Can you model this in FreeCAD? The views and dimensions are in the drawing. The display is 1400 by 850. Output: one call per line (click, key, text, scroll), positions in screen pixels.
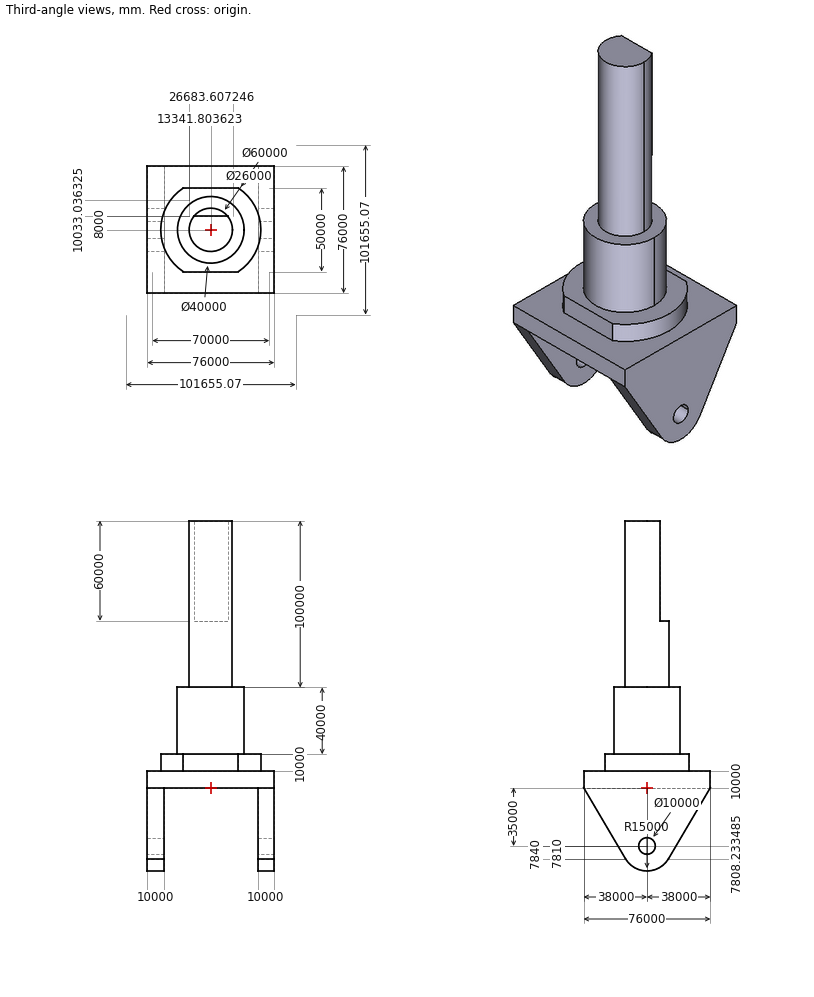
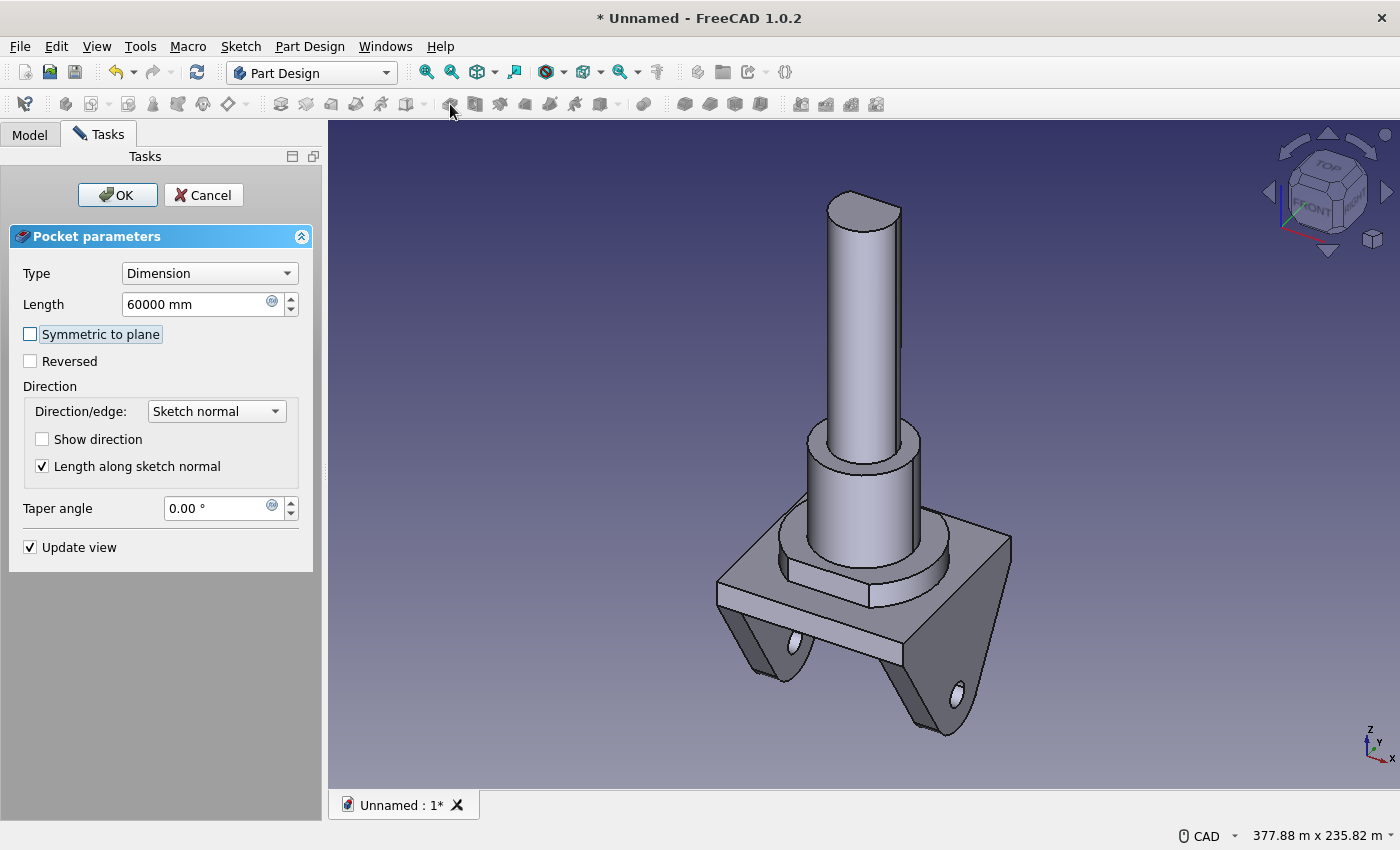
click(118, 195)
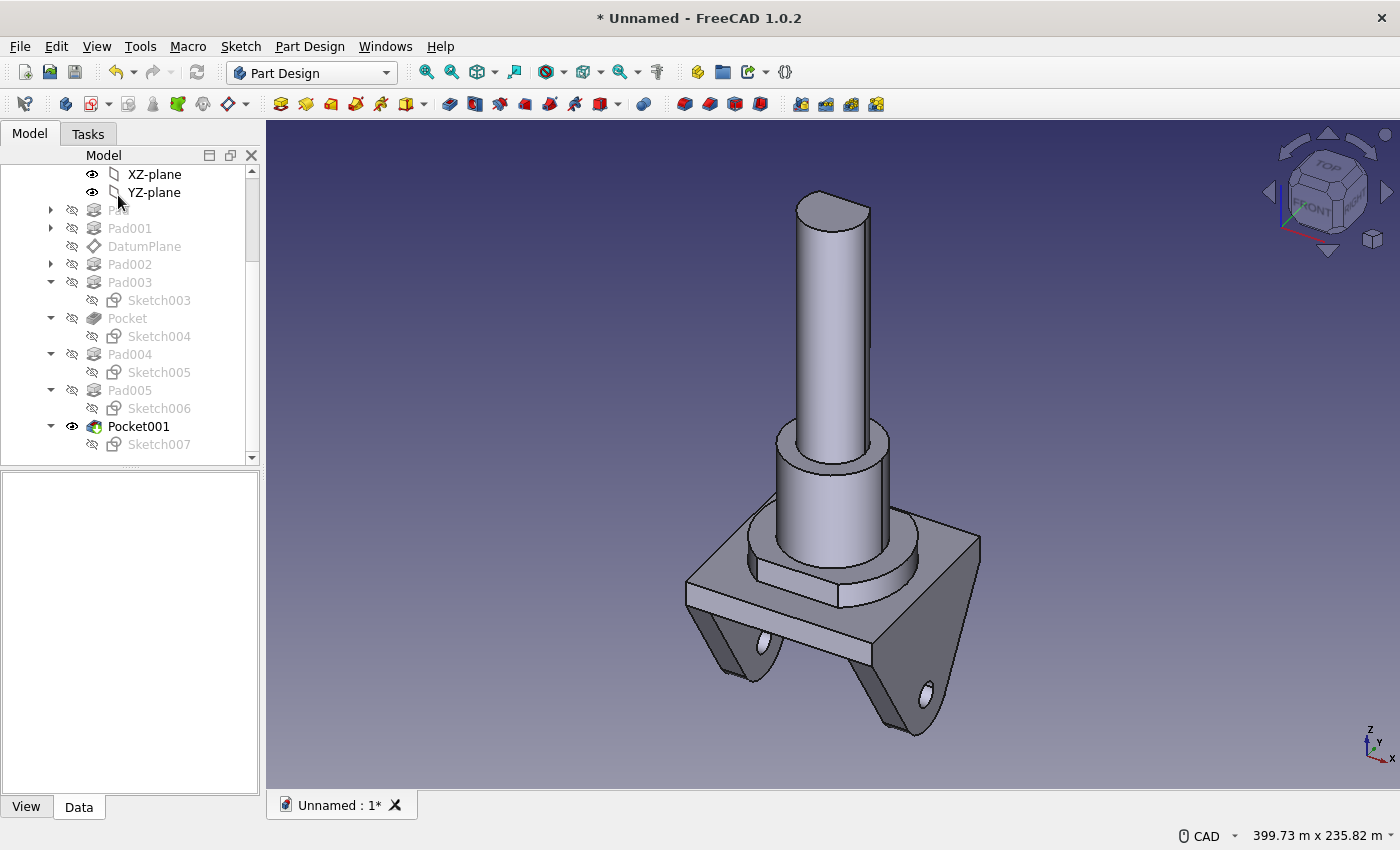
key(0)